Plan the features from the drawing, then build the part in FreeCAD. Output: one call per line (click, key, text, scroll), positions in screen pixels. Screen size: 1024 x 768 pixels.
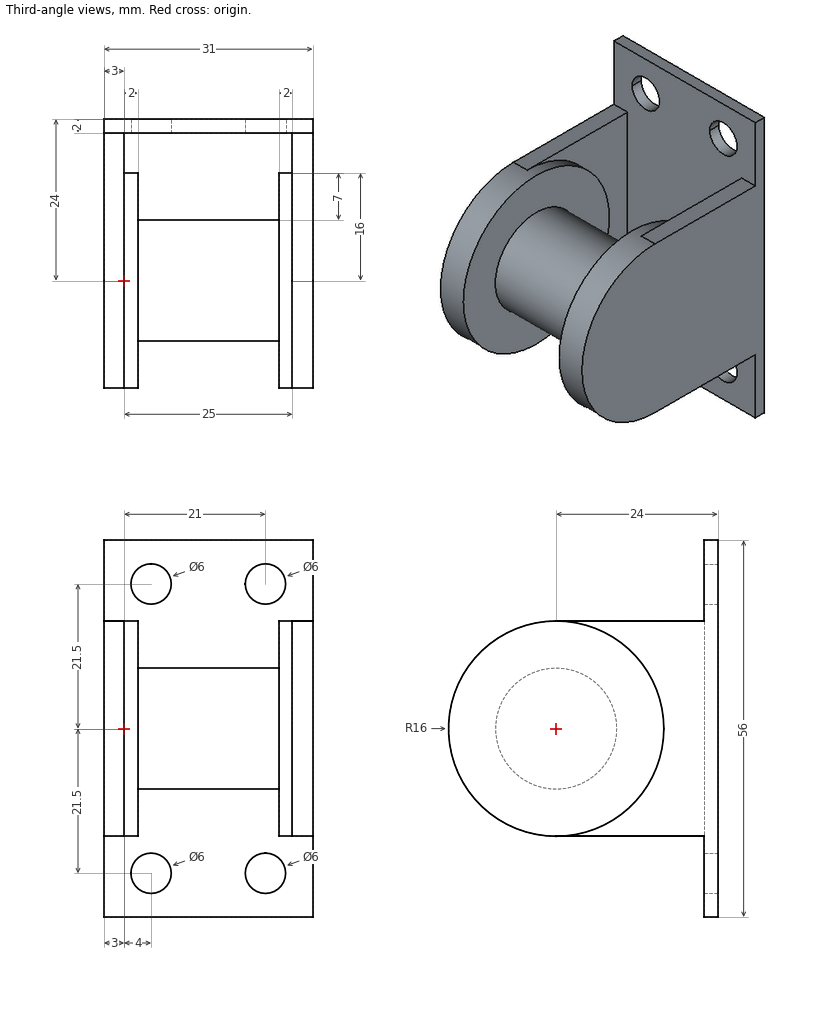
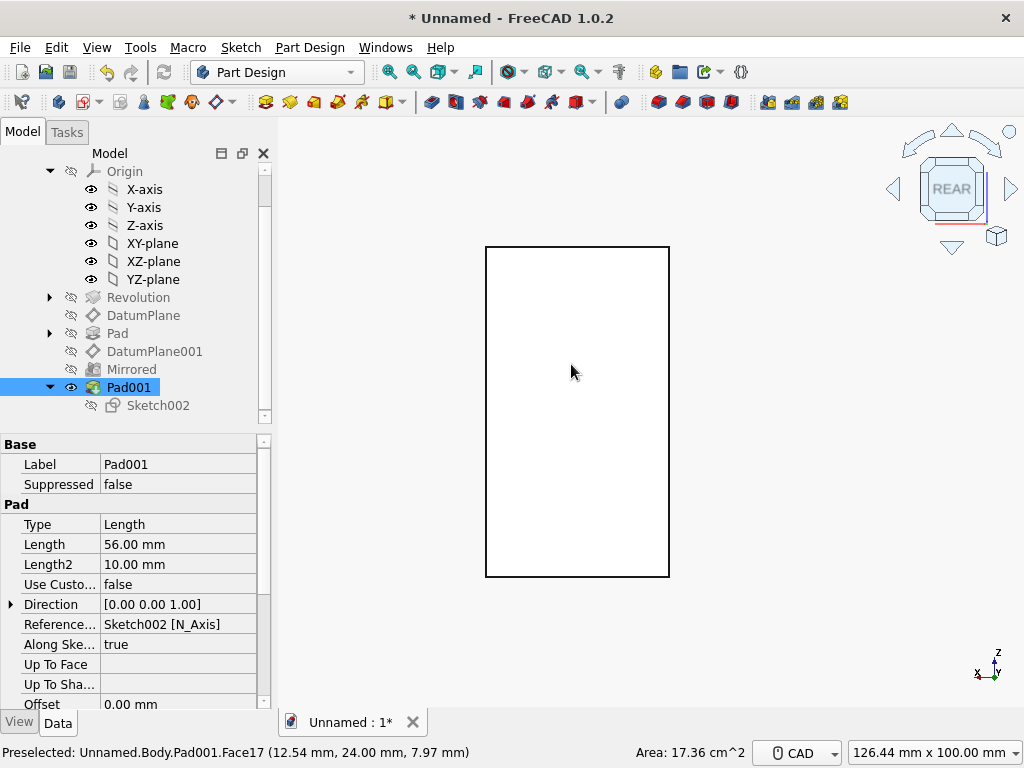
click(84, 102)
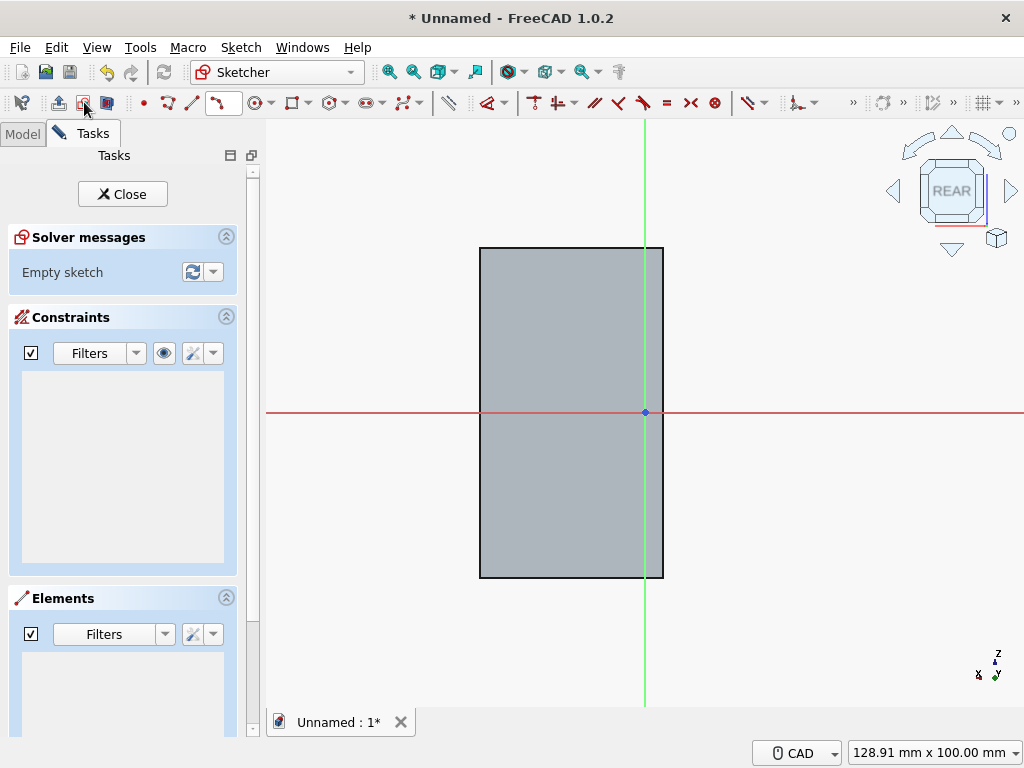
scroll(626, 552, up, 12)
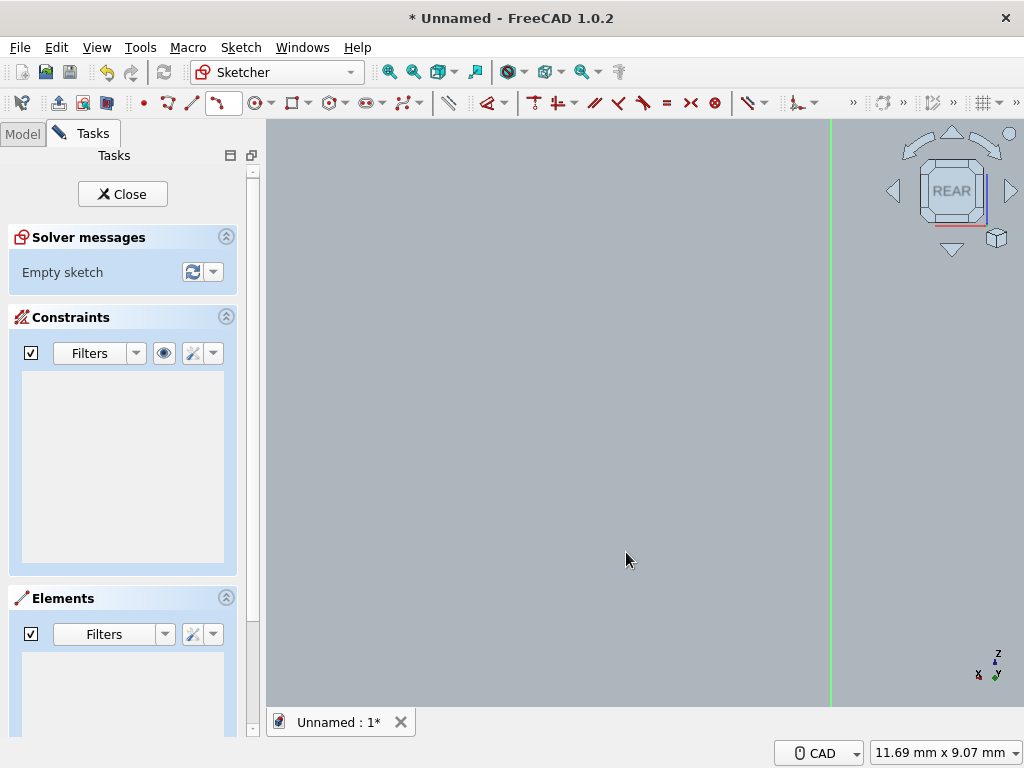
click(256, 104)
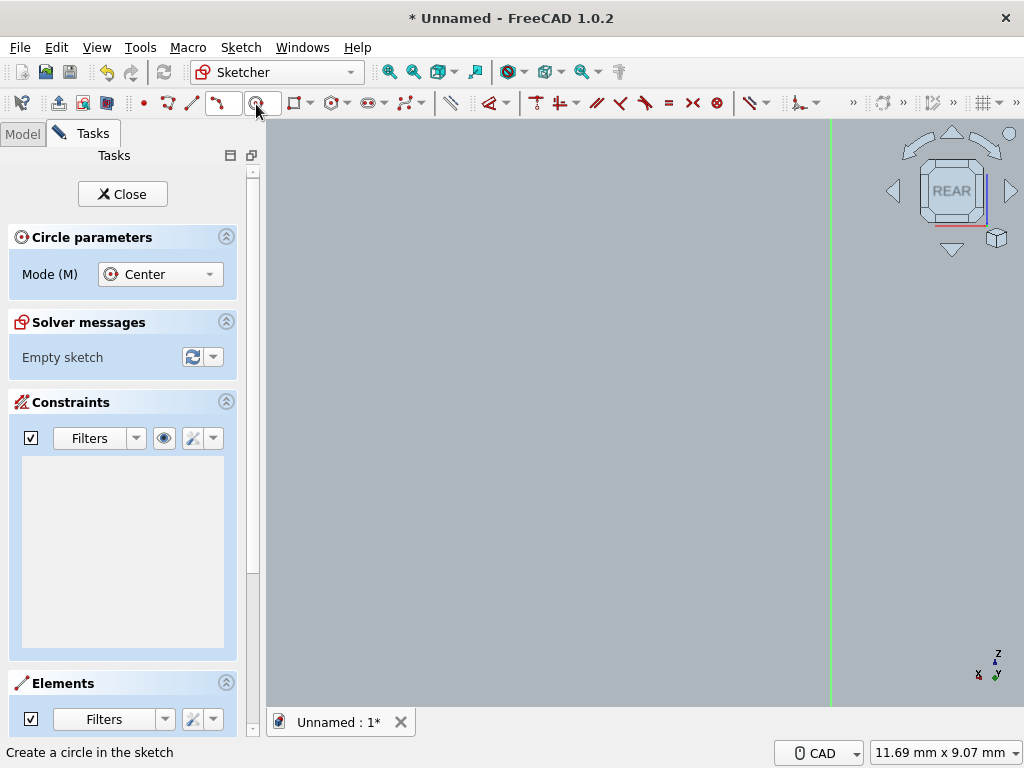
click(571, 406)
click(709, 268)
key(Escape)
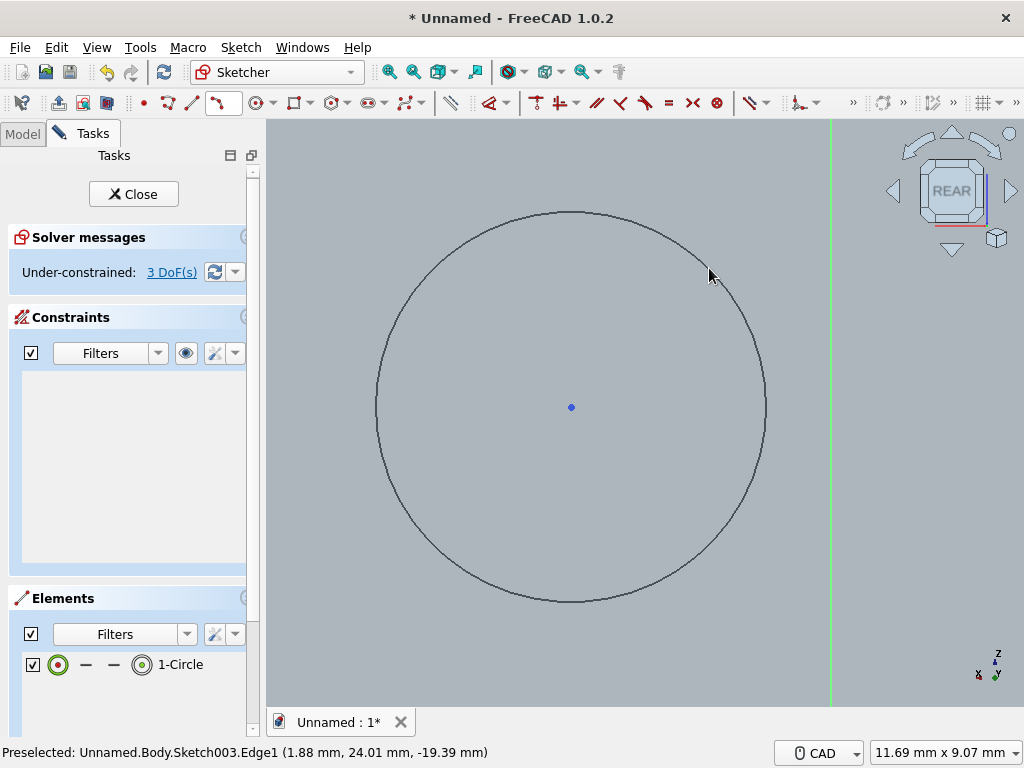
click(490, 104)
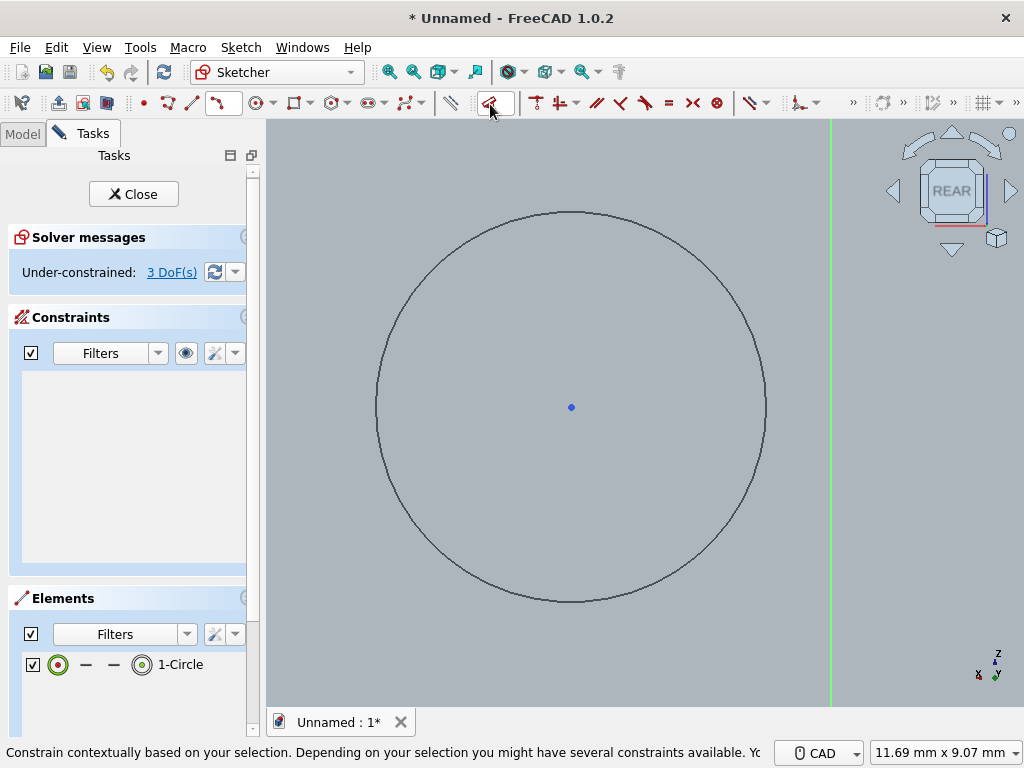
click(709, 269)
click(732, 246)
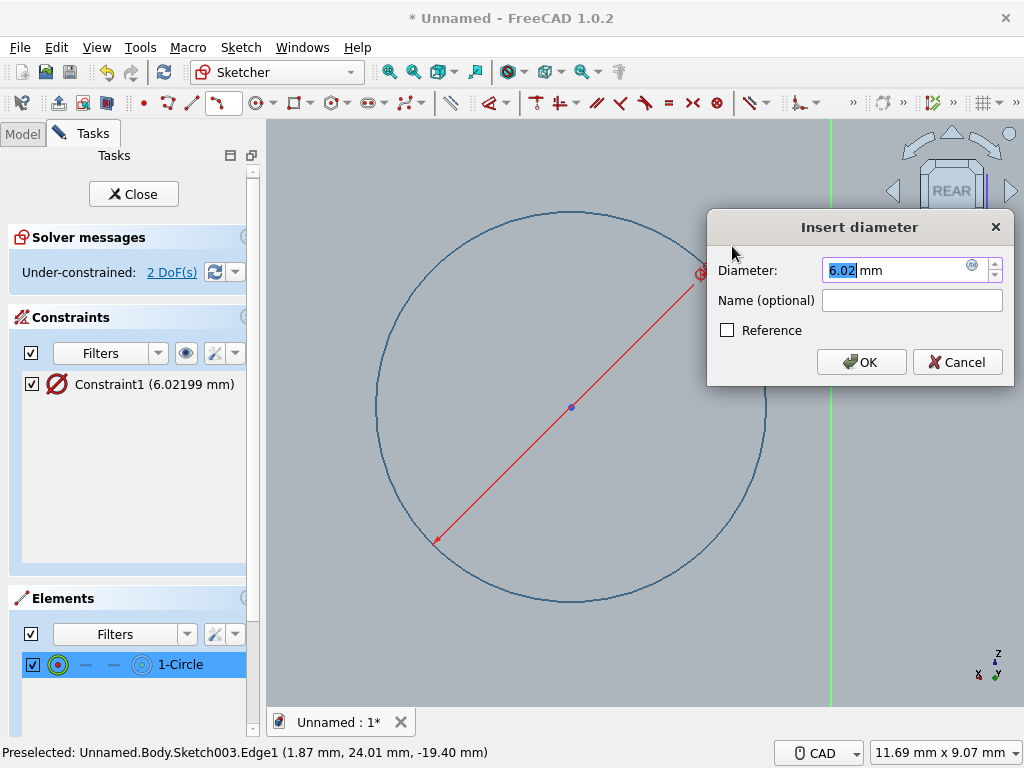
text(6)
key(Return)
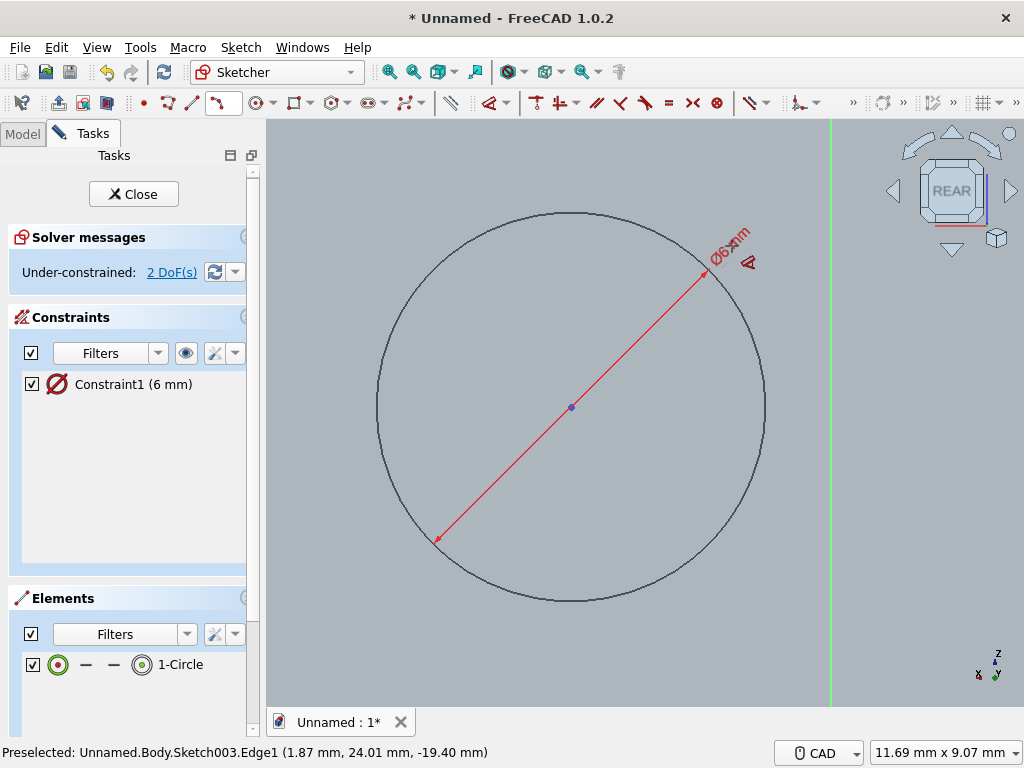
click(571, 407)
click(701, 441)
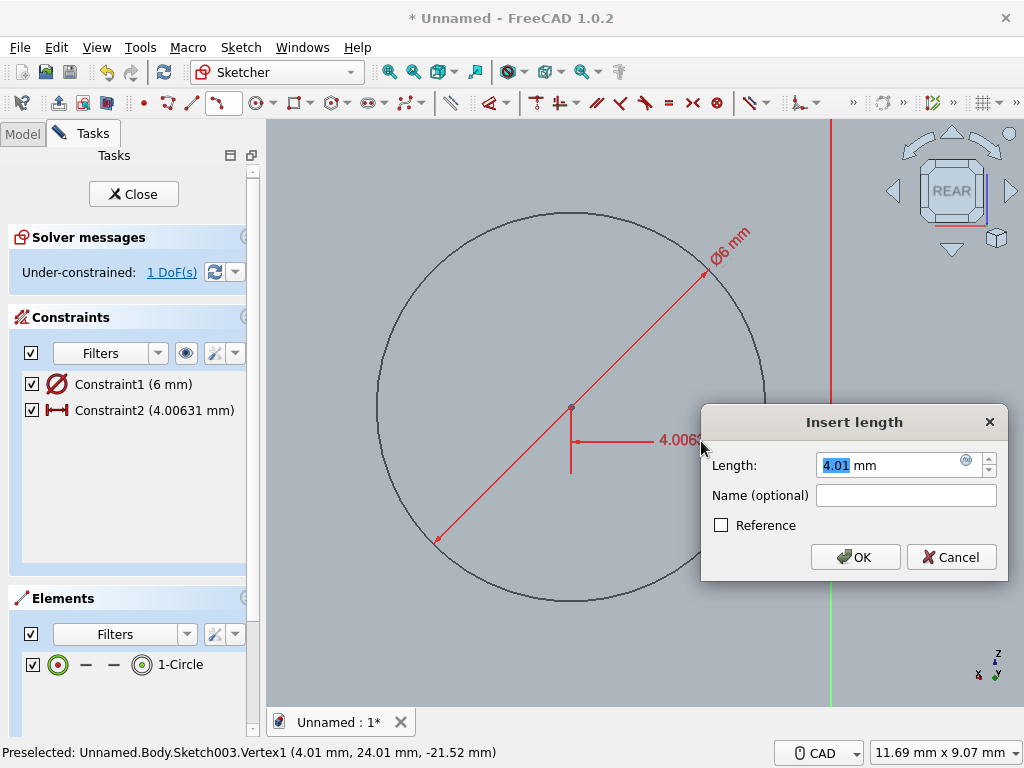
text(4)
key(Return)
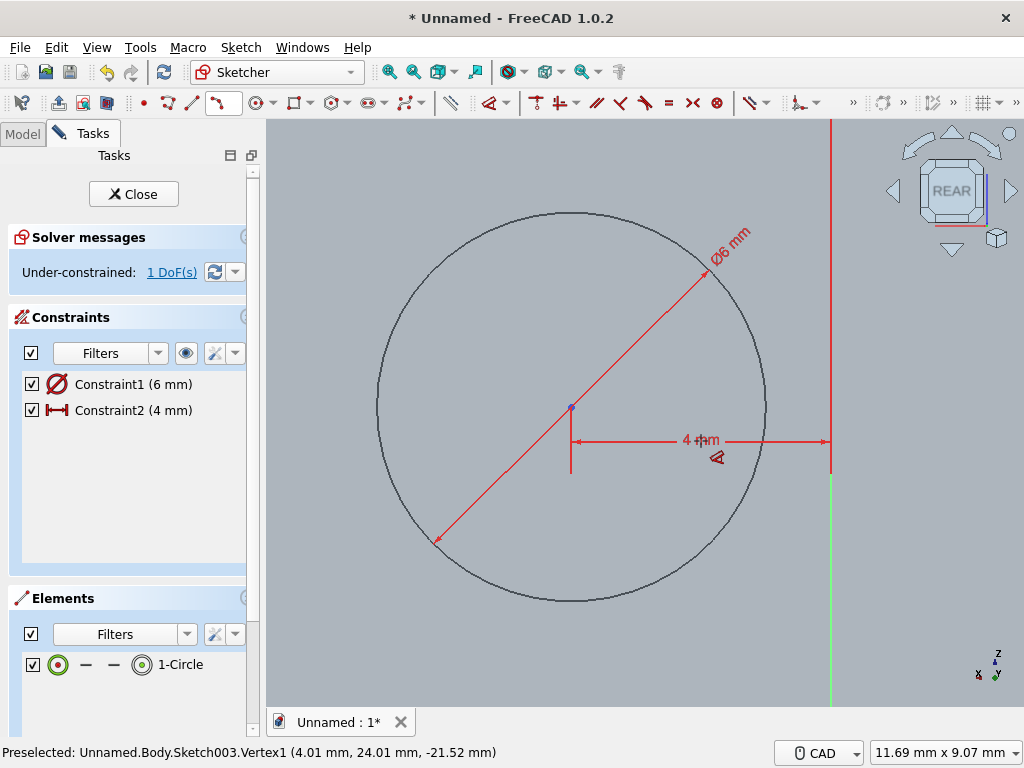
click(571, 407)
click(537, 277)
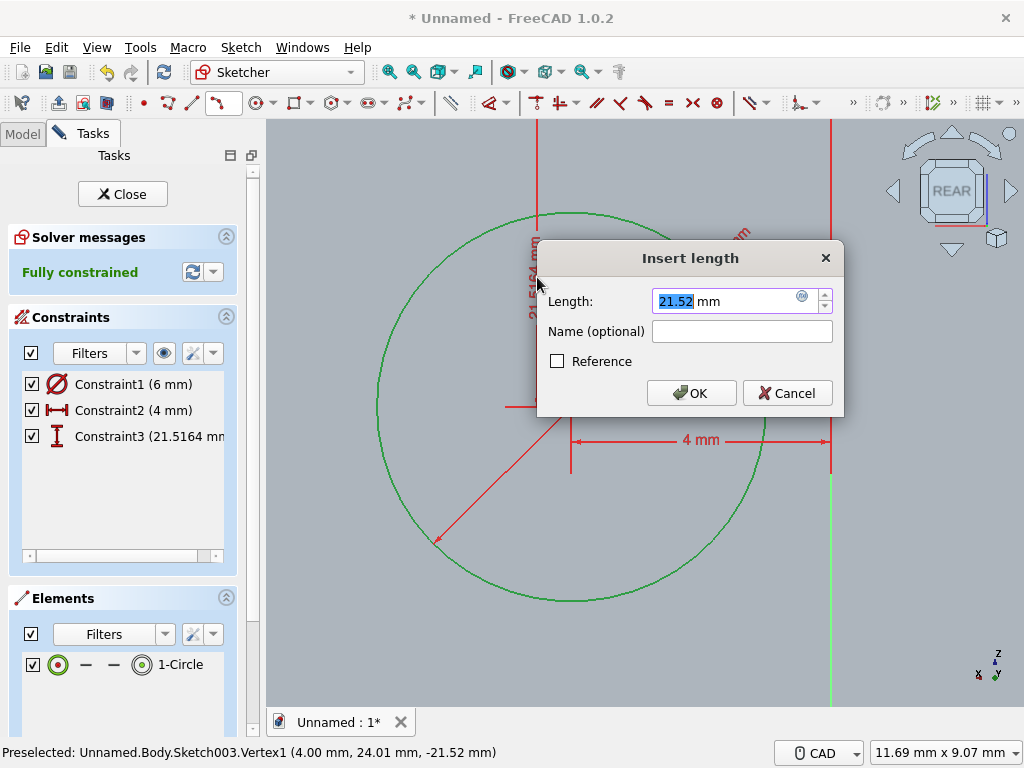
text(21.5)
key(Return)
key(Escape)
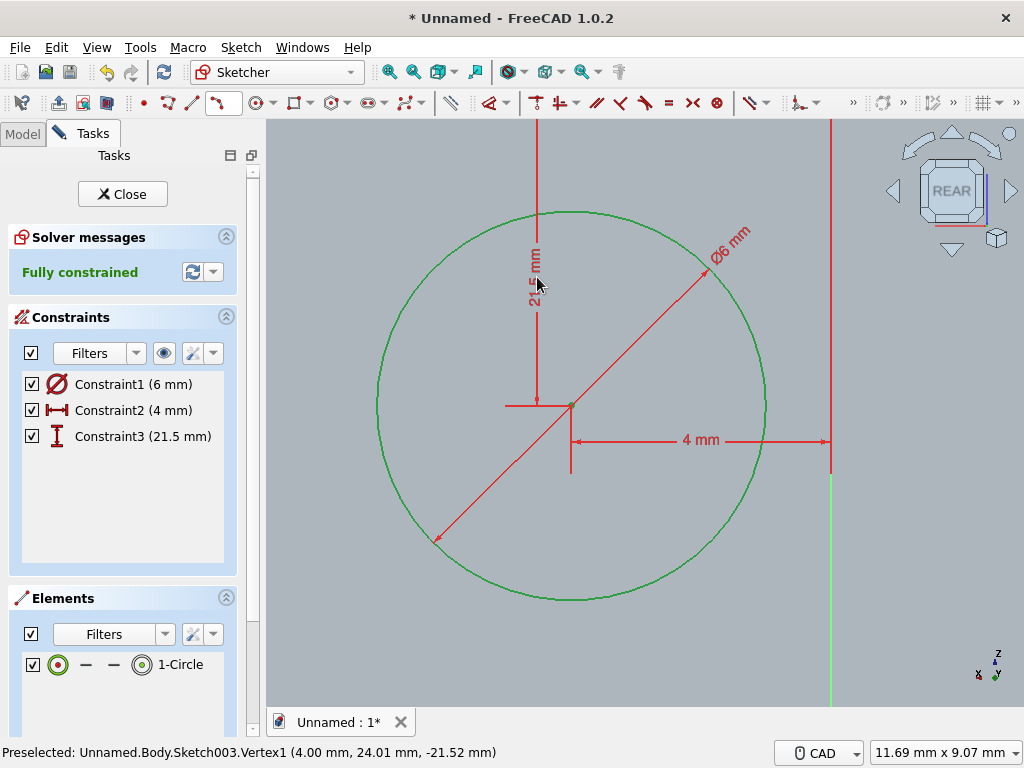
click(123, 194)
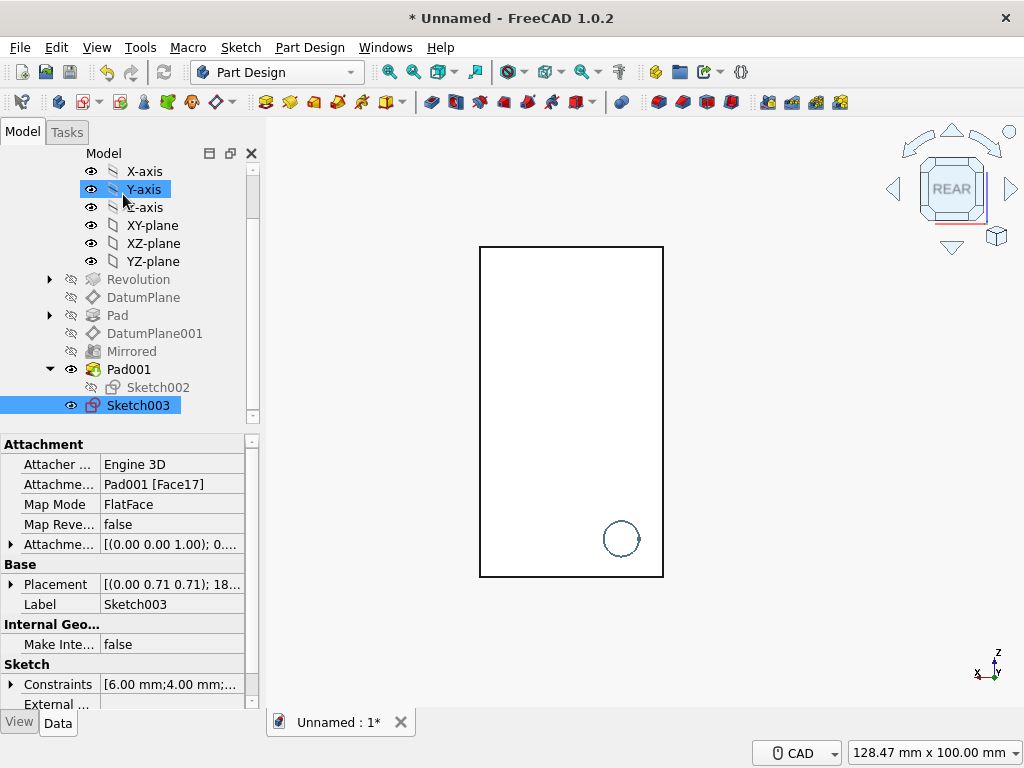
click(432, 102)